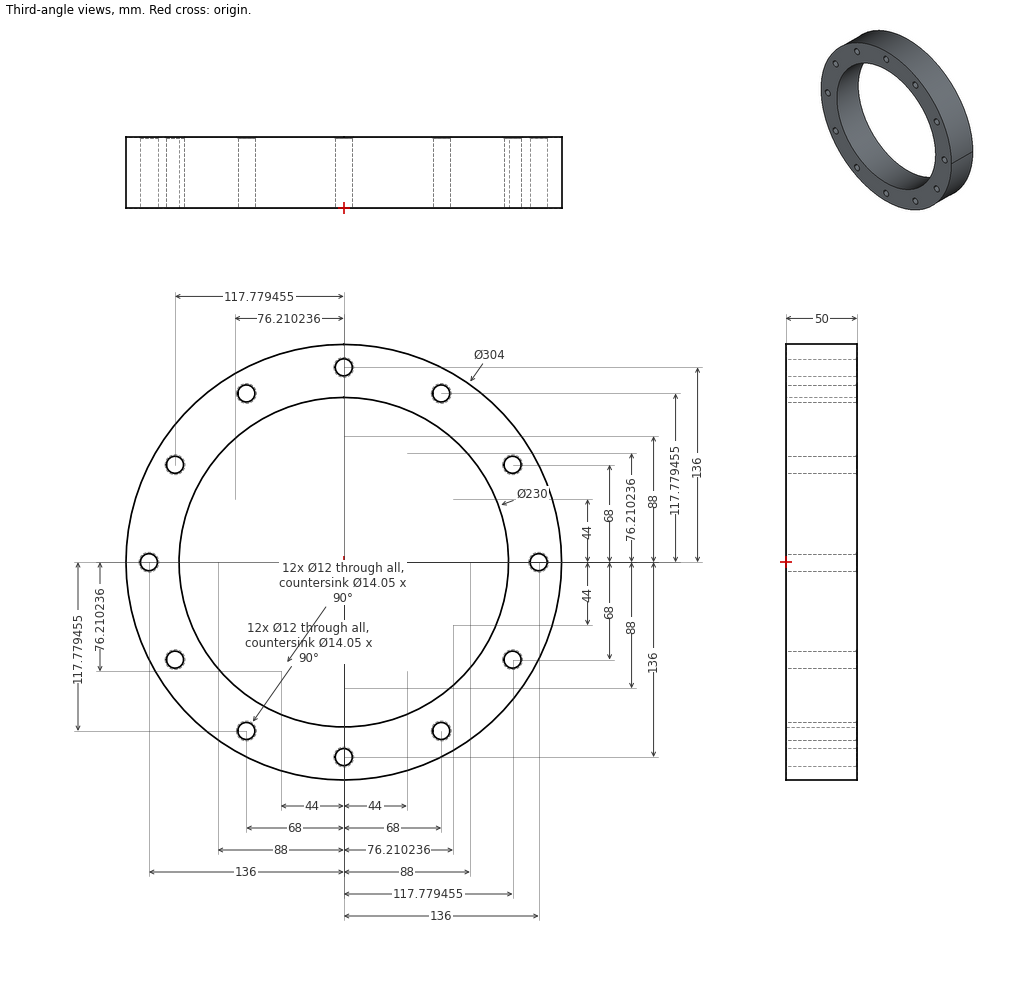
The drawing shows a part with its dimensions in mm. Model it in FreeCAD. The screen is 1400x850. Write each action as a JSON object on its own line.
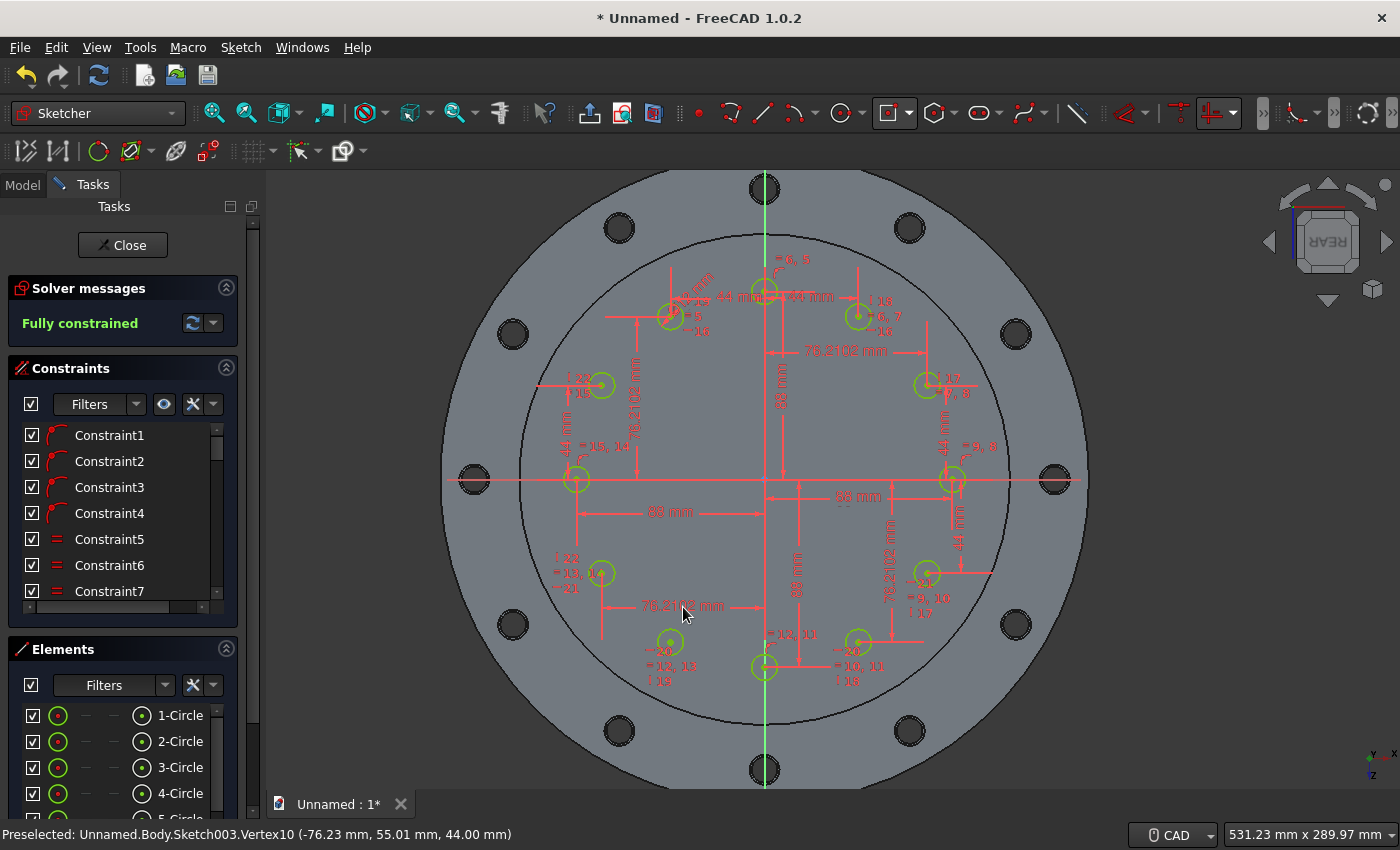
{"action": "left_click", "coordinate": [123, 245]}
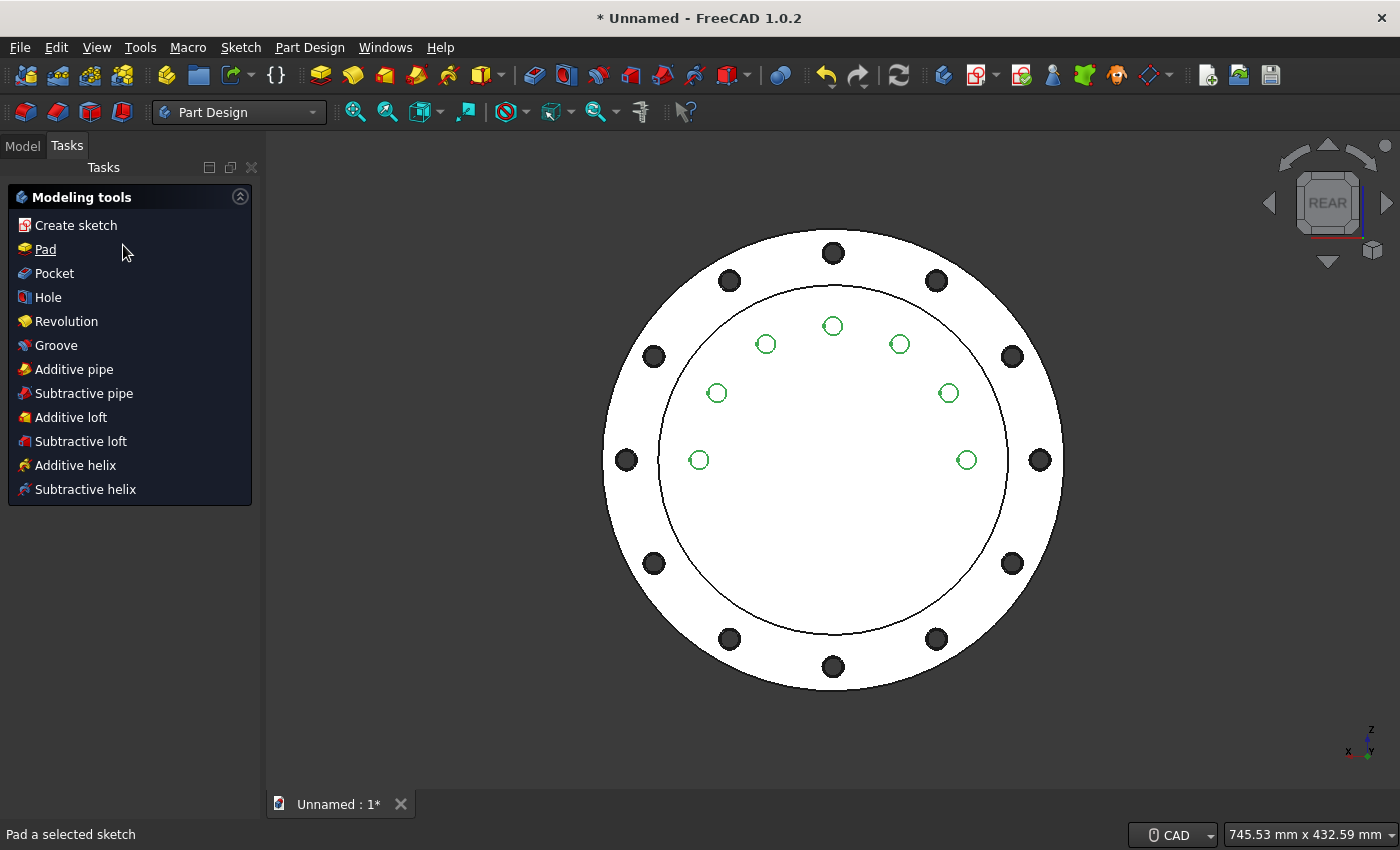
{"action": "left_click", "coordinate": [568, 76]}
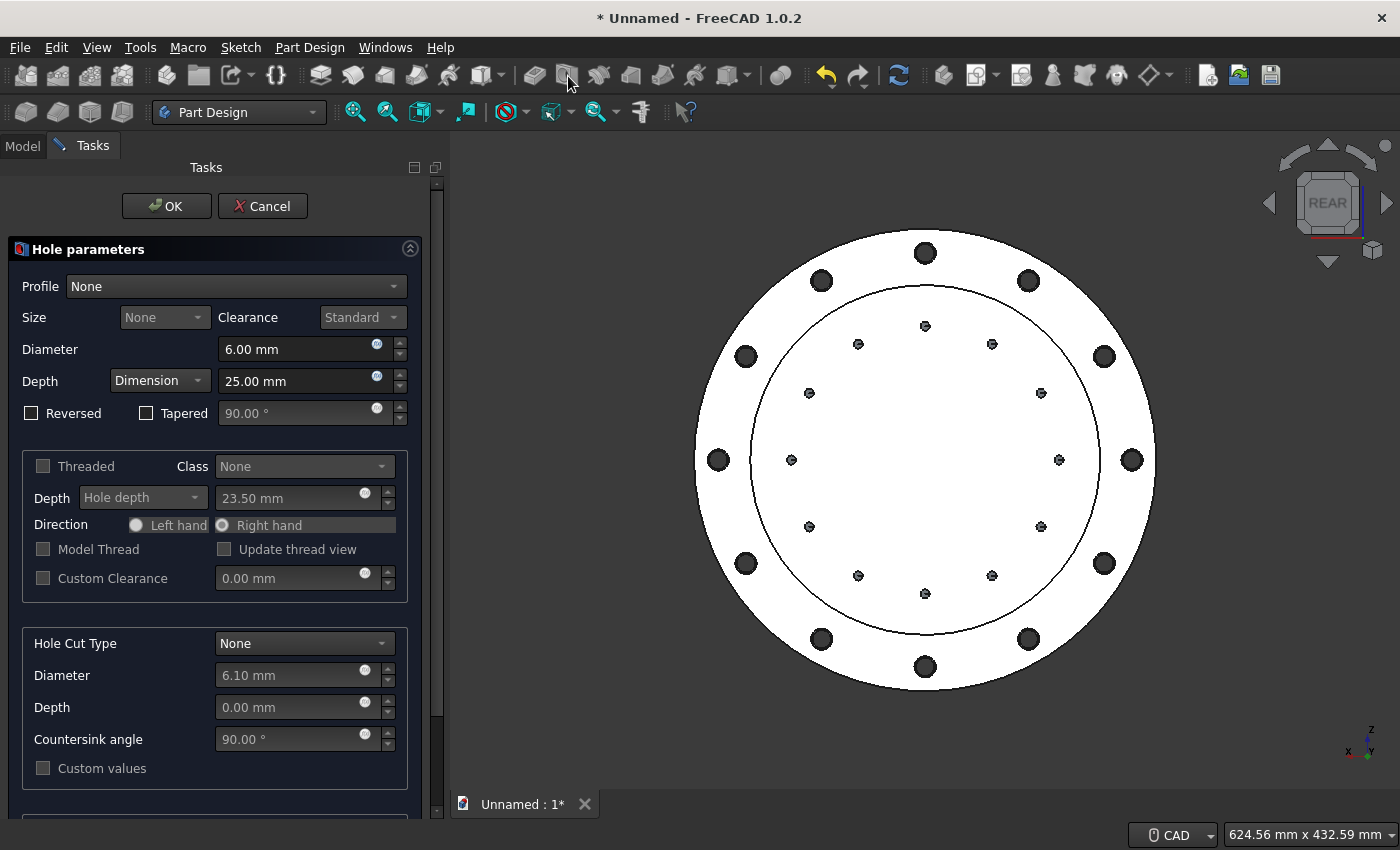
{"action": "triple_click", "coordinate": [305, 349]}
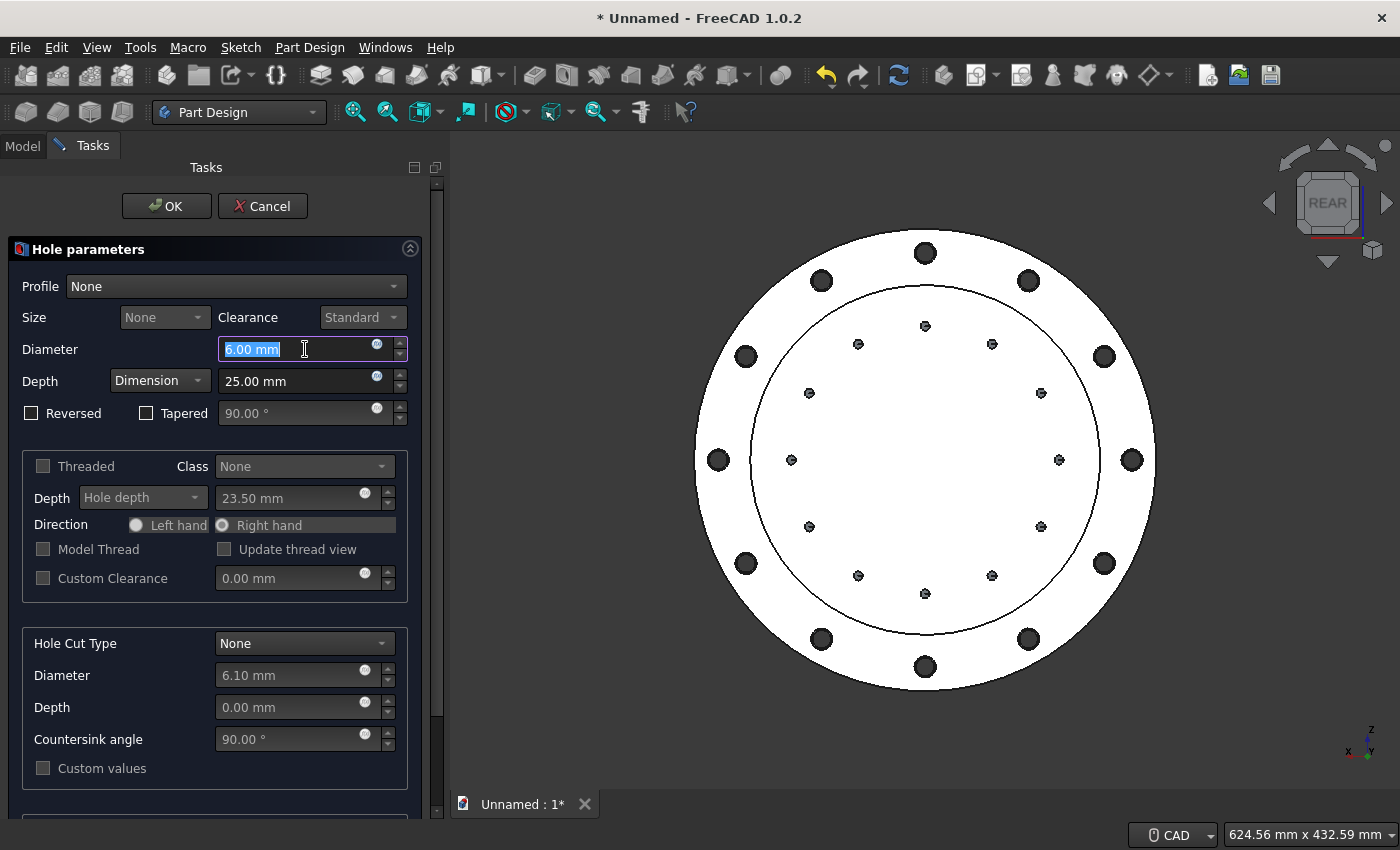
{"action": "type", "text": "12"}
{"action": "key", "text": "Tab"}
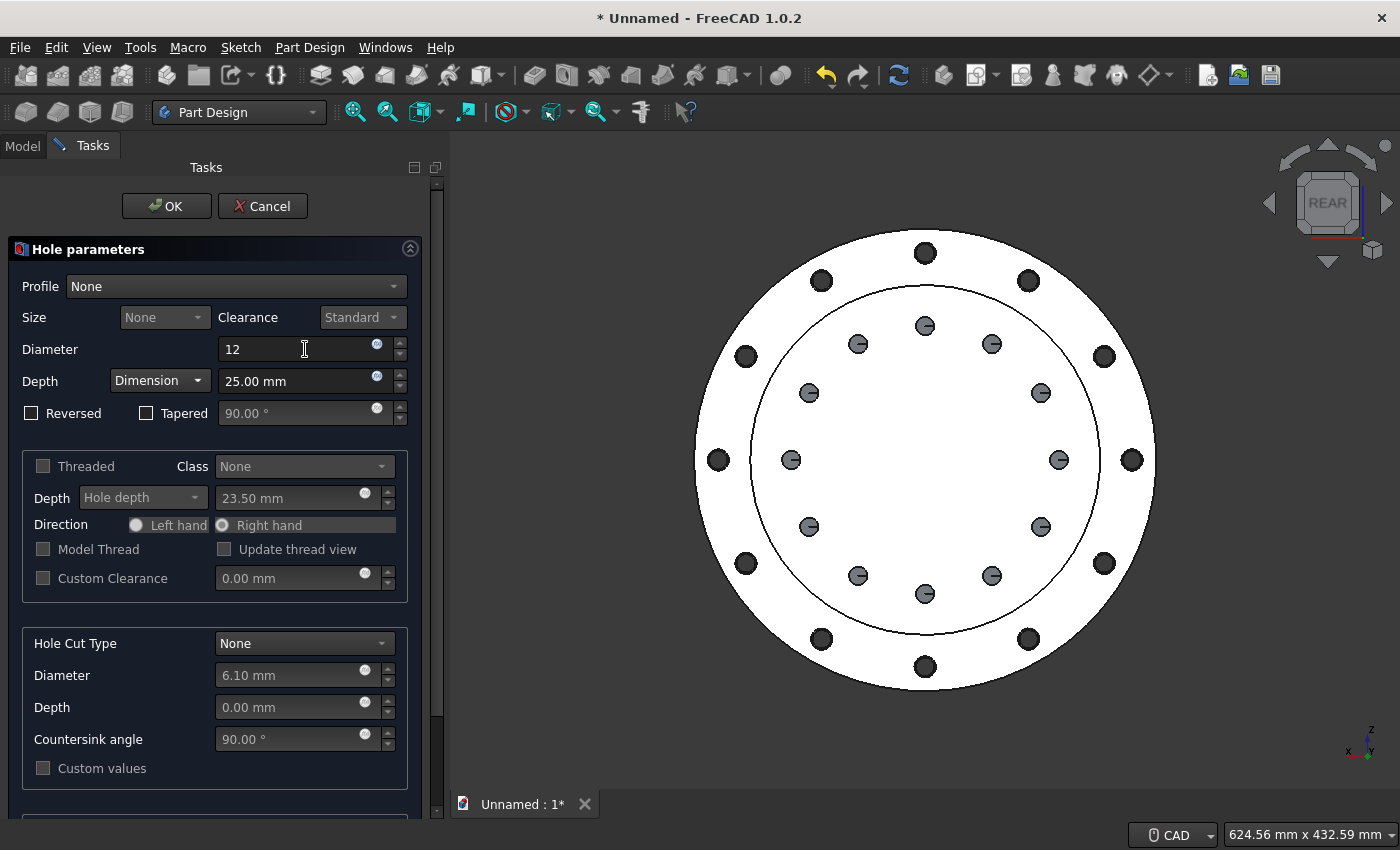
{"action": "left_click", "coordinate": [161, 380]}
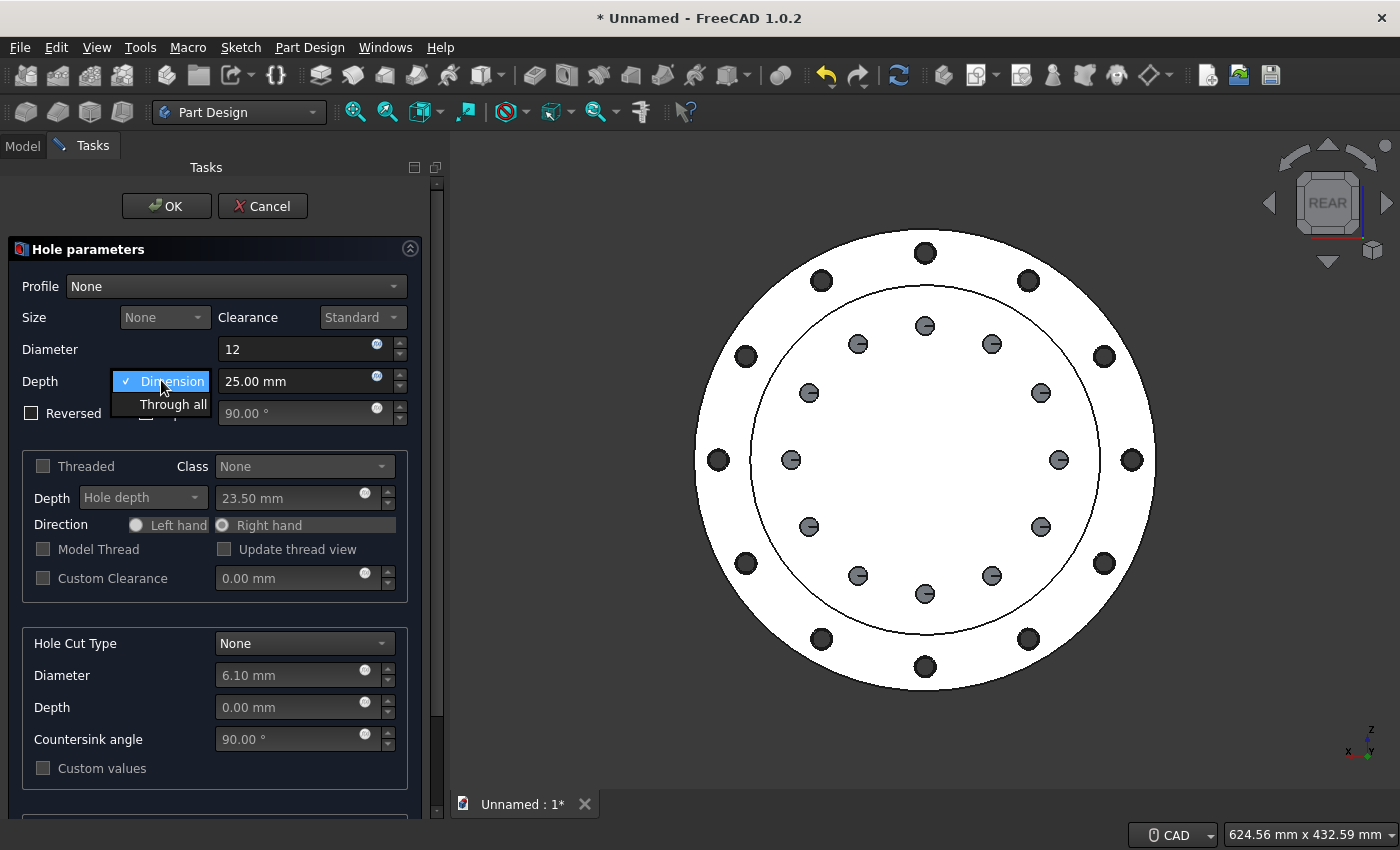
{"action": "left_click", "coordinate": [160, 404]}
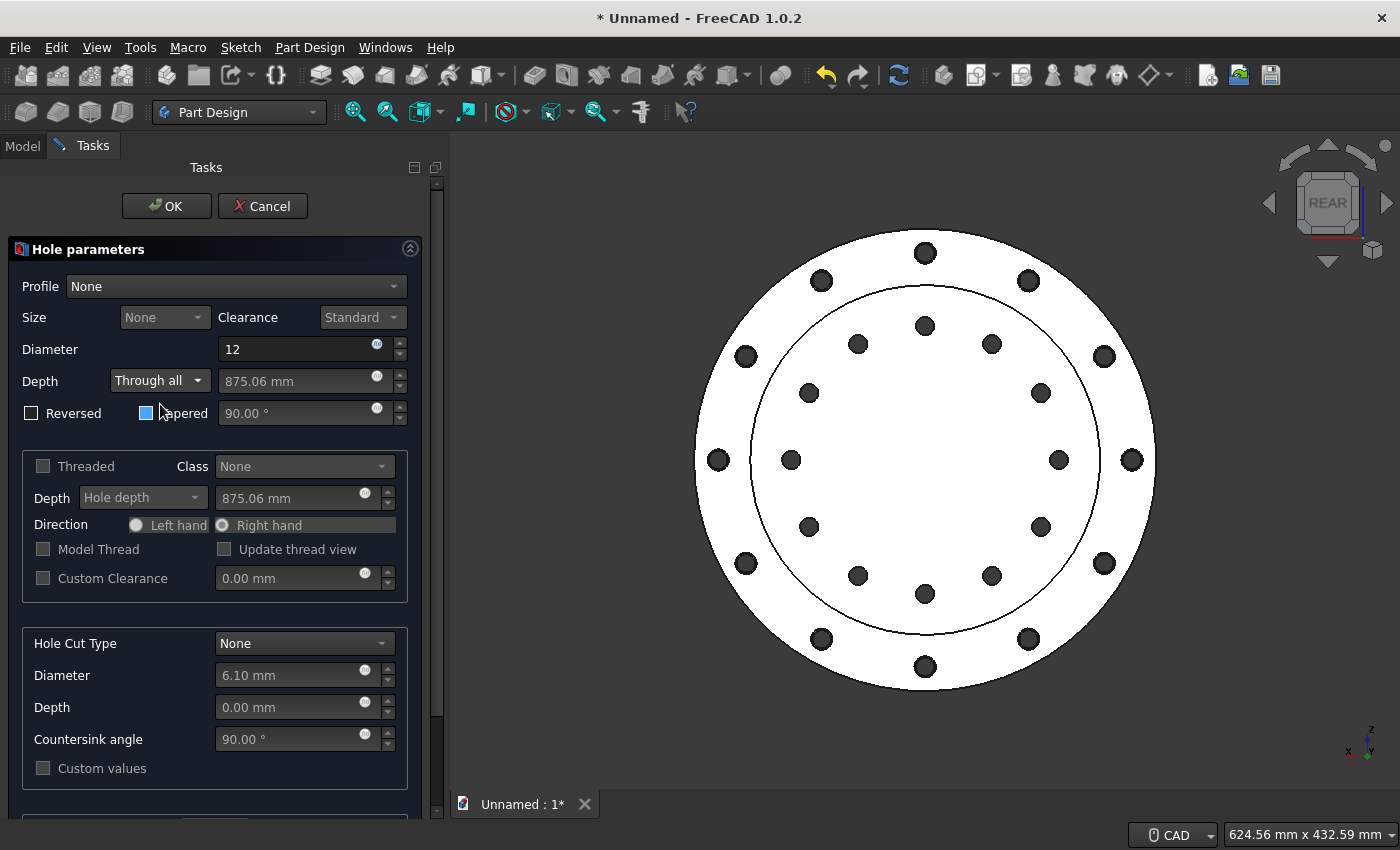
{"action": "left_click", "coordinate": [306, 644]}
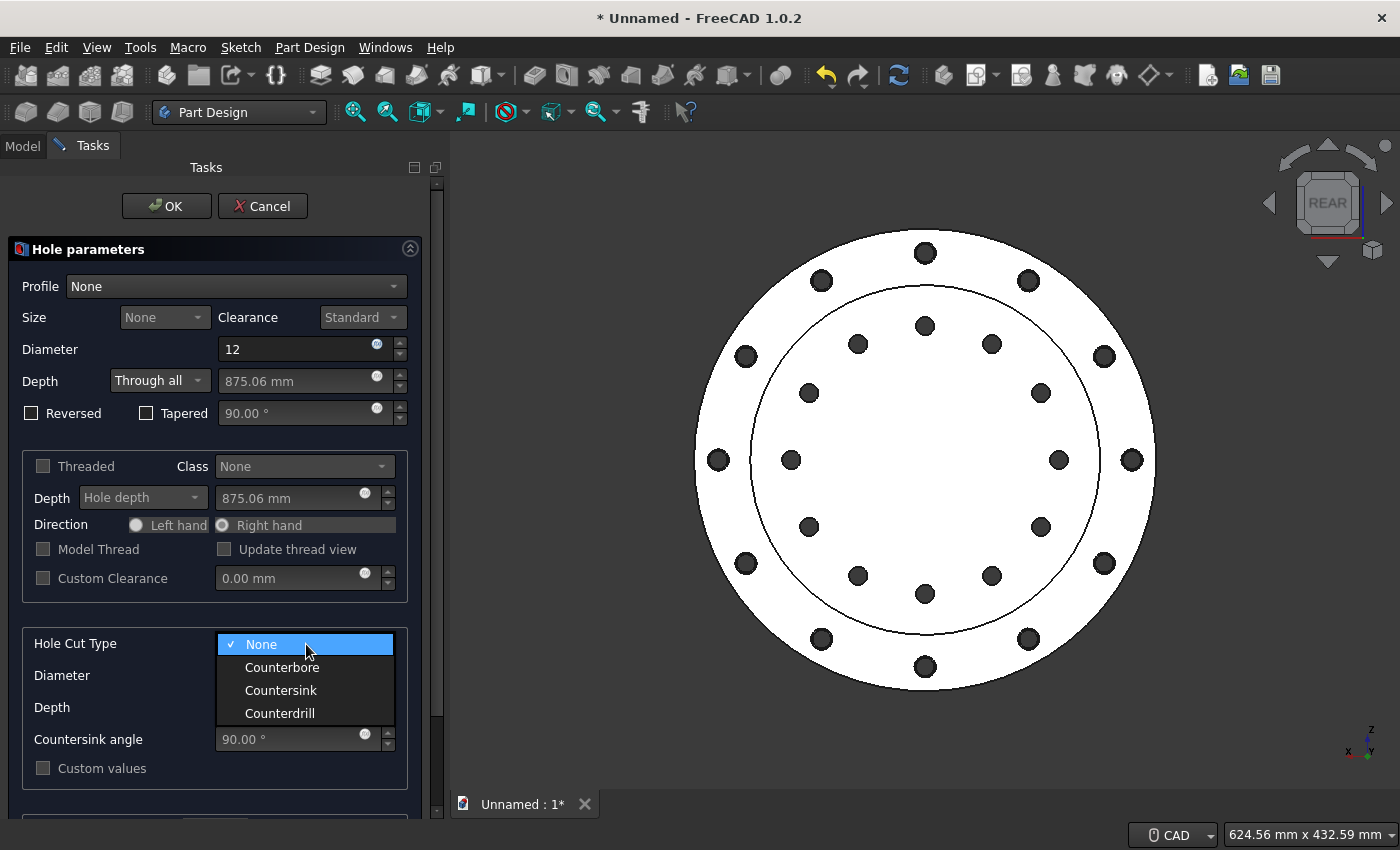
{"action": "left_click", "coordinate": [304, 690]}